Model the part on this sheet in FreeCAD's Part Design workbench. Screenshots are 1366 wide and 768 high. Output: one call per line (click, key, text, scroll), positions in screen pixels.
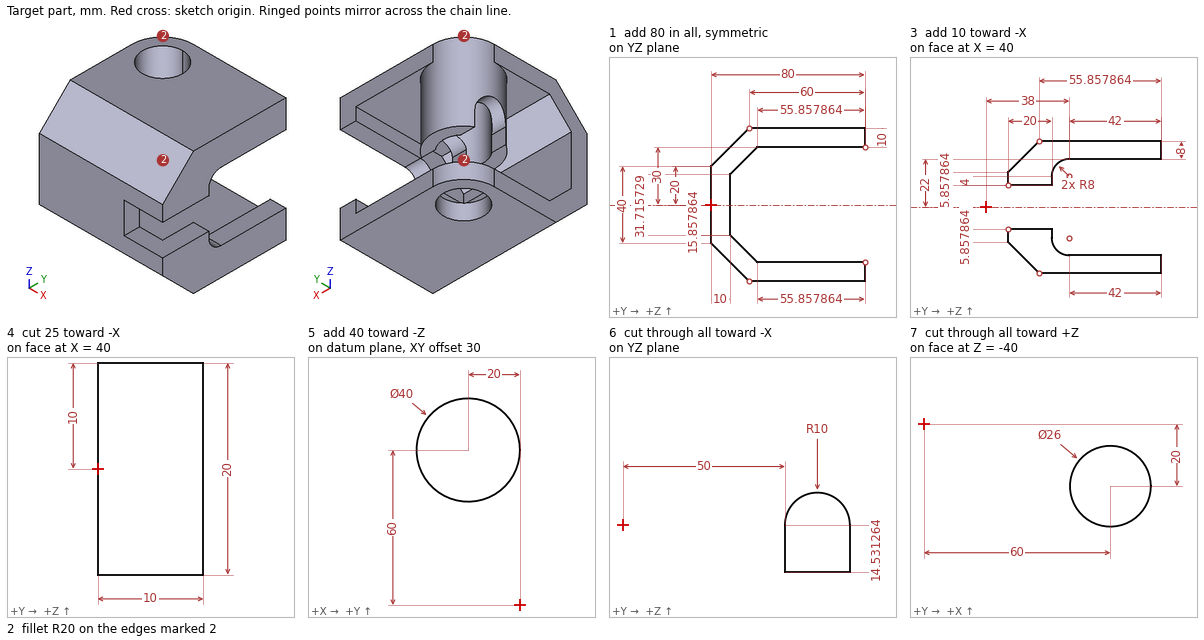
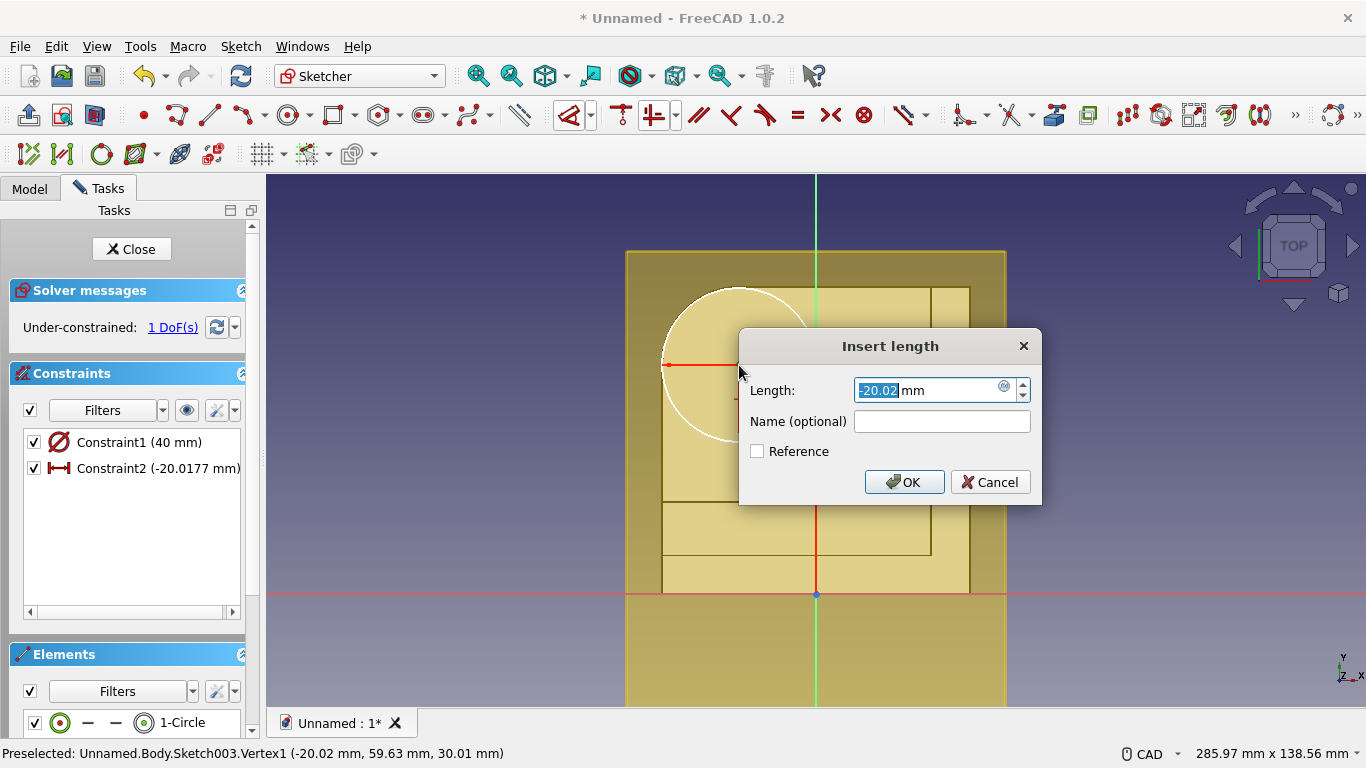
text(-20)
key(Return)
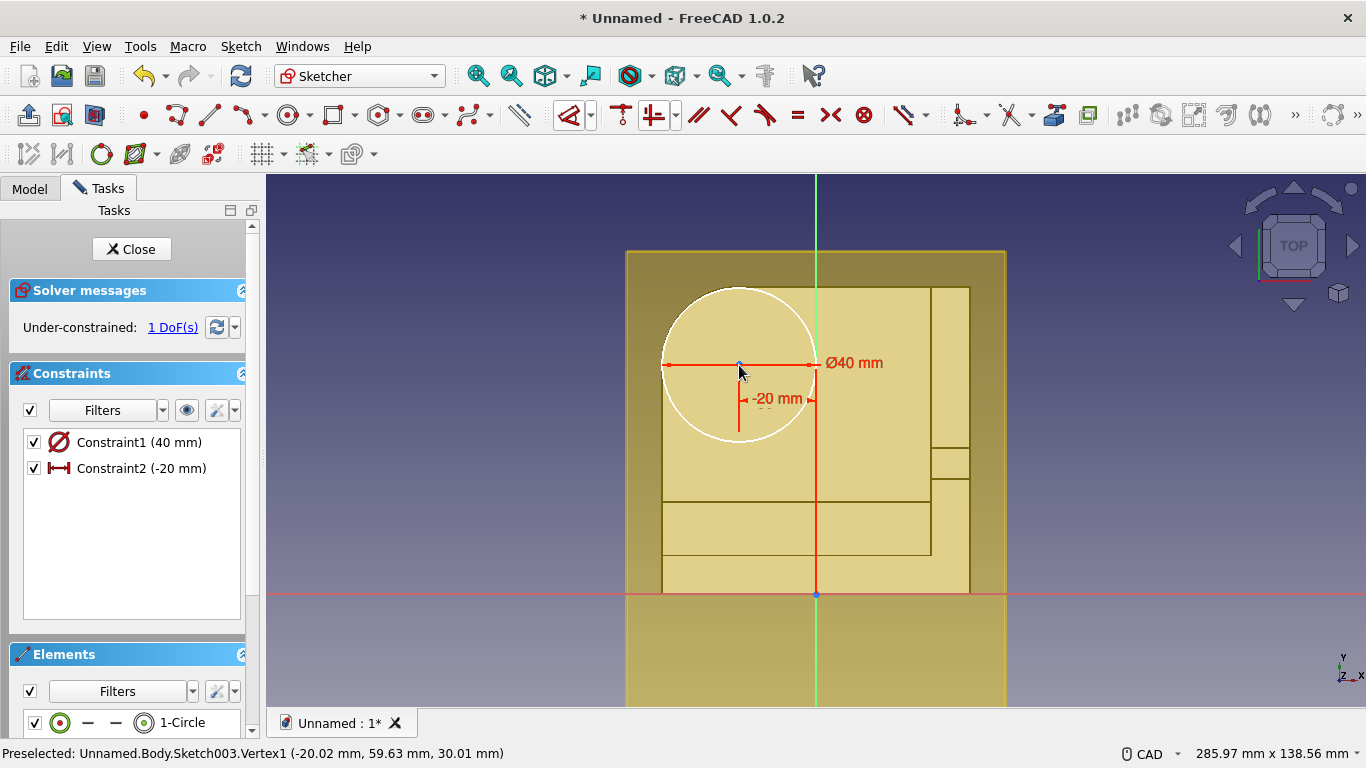
click(739, 365)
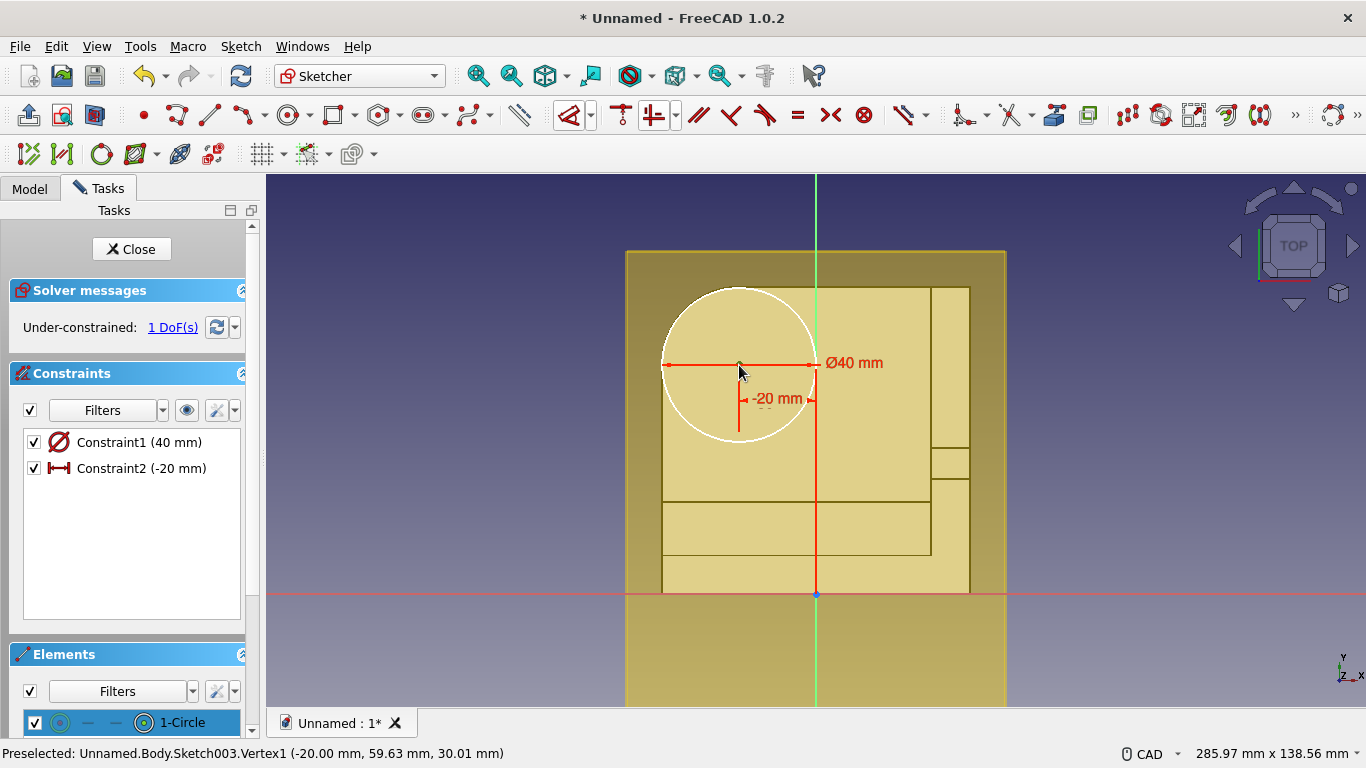
click(590, 116)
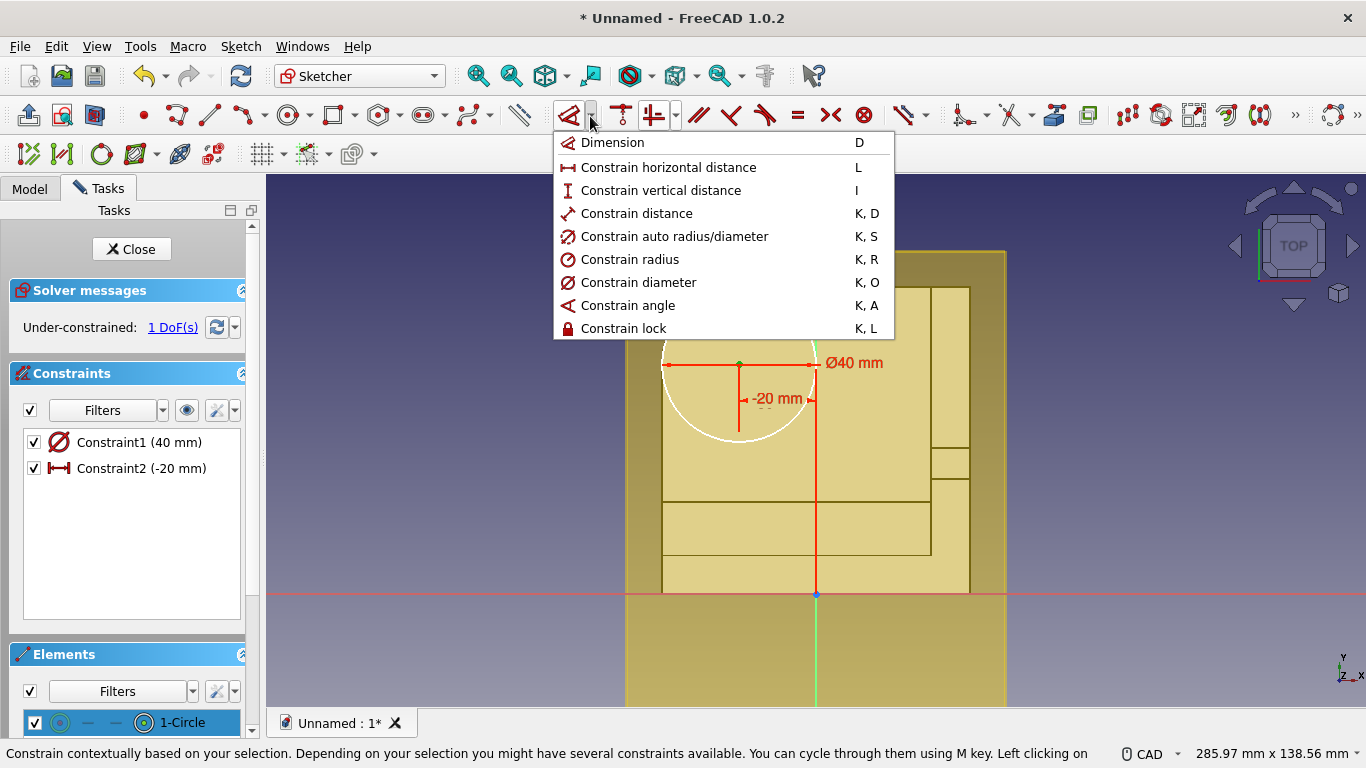
click(724, 190)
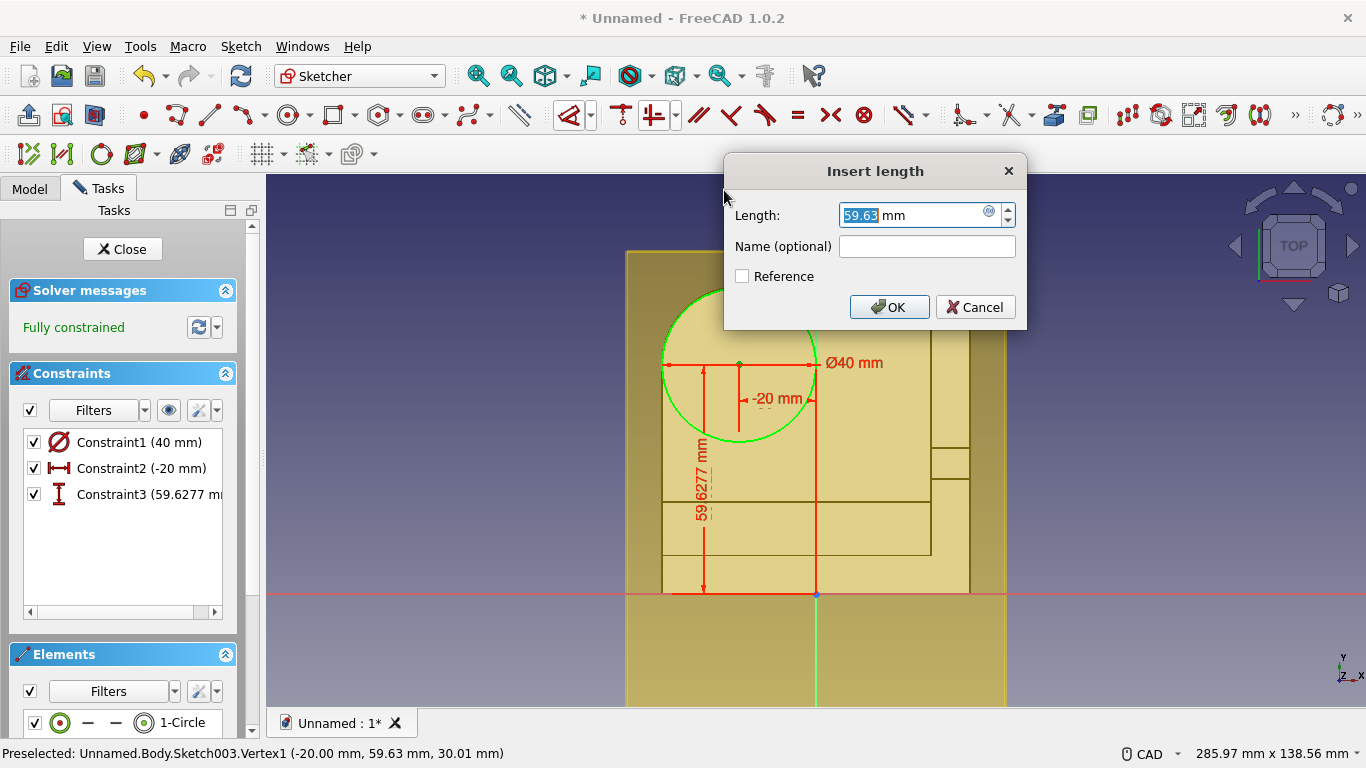
text(60)
key(Return)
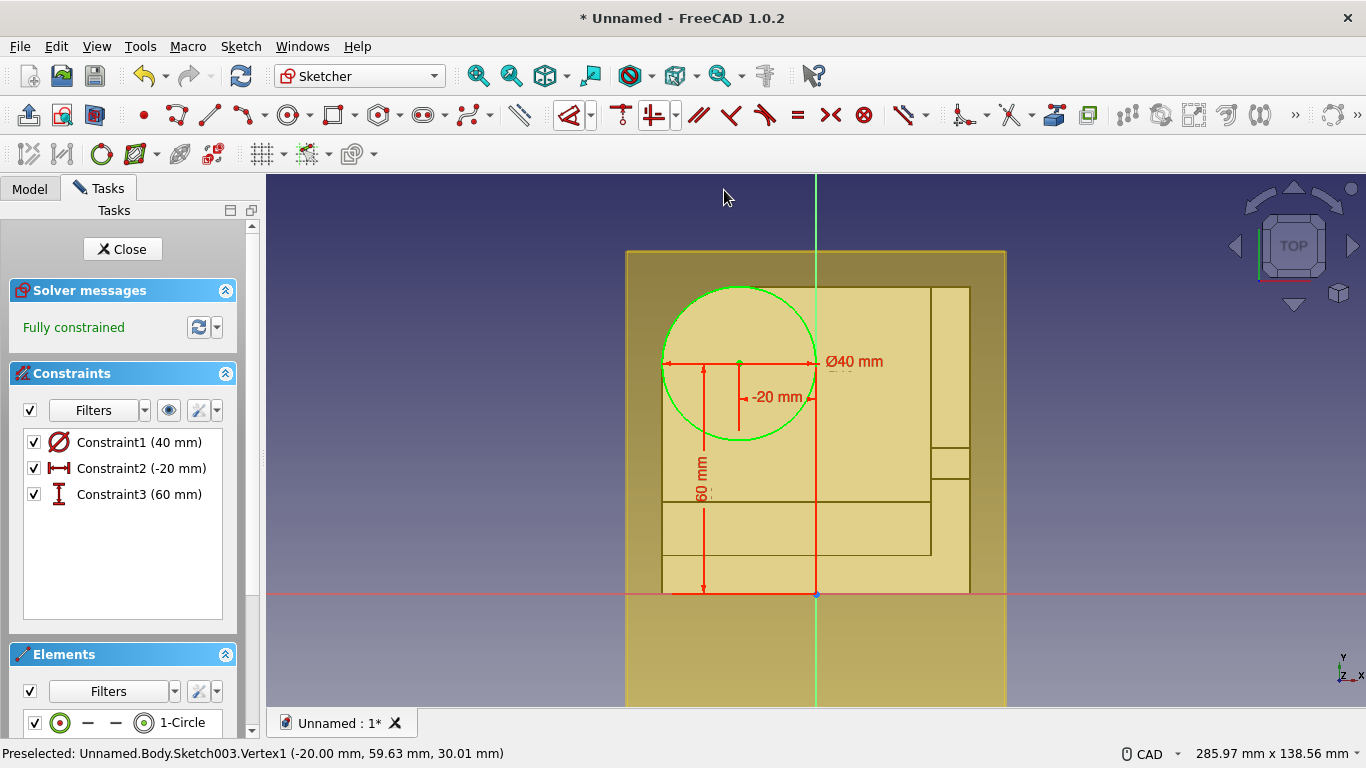
click(123, 249)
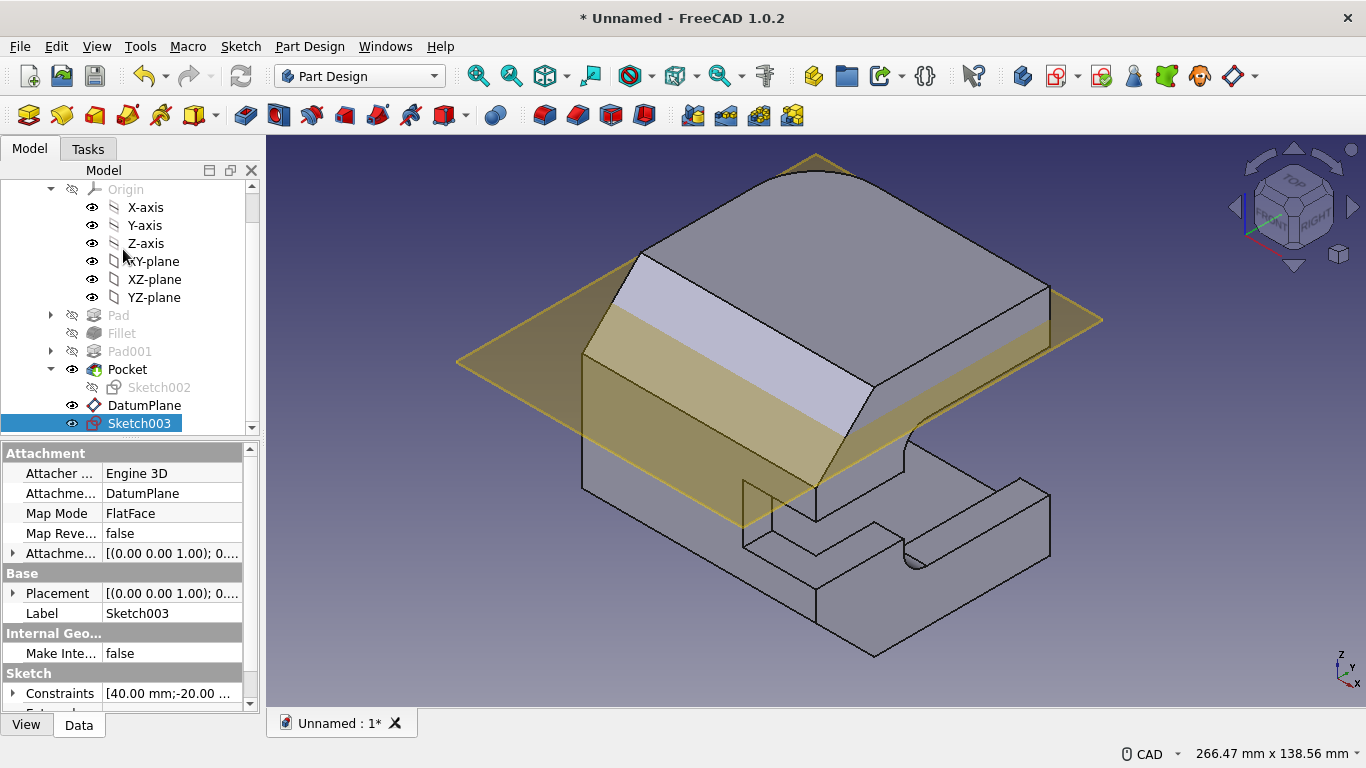
click(29, 116)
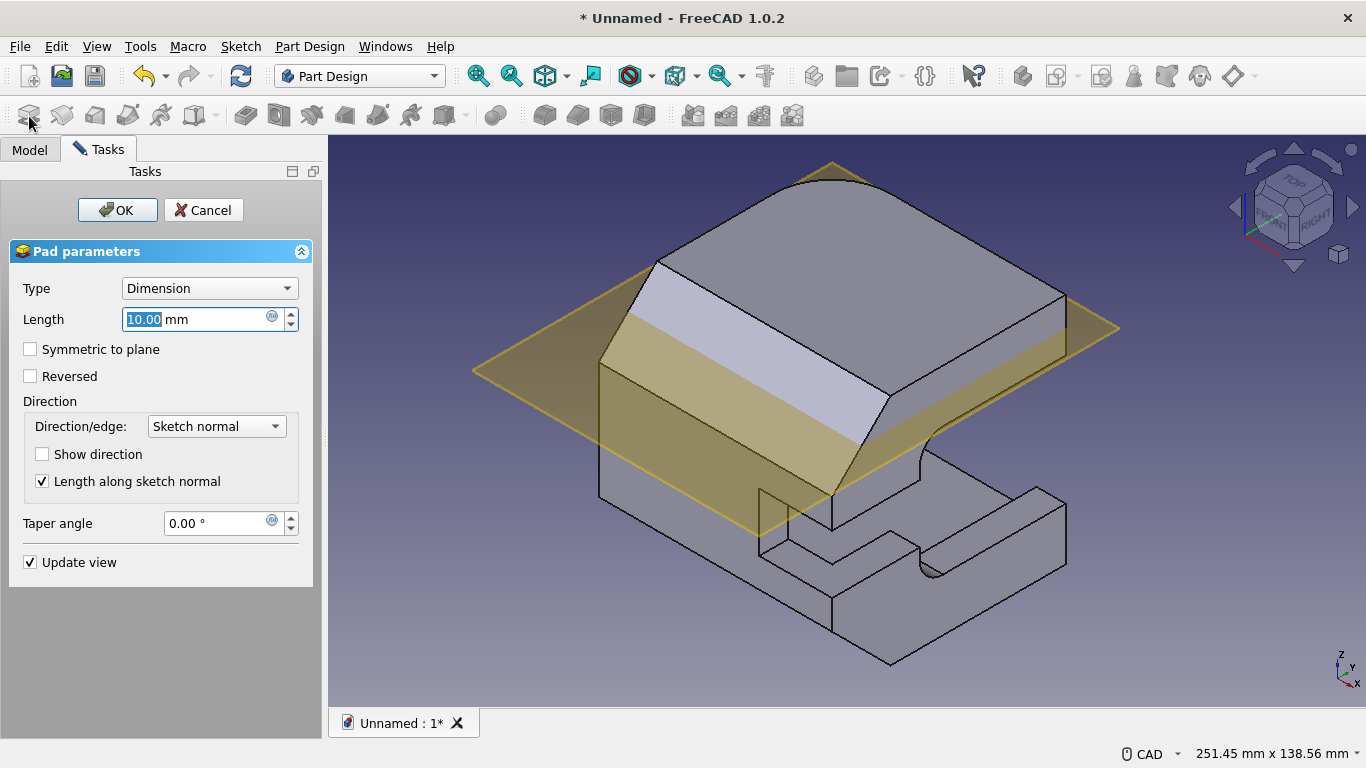
text(40)
key(Tab)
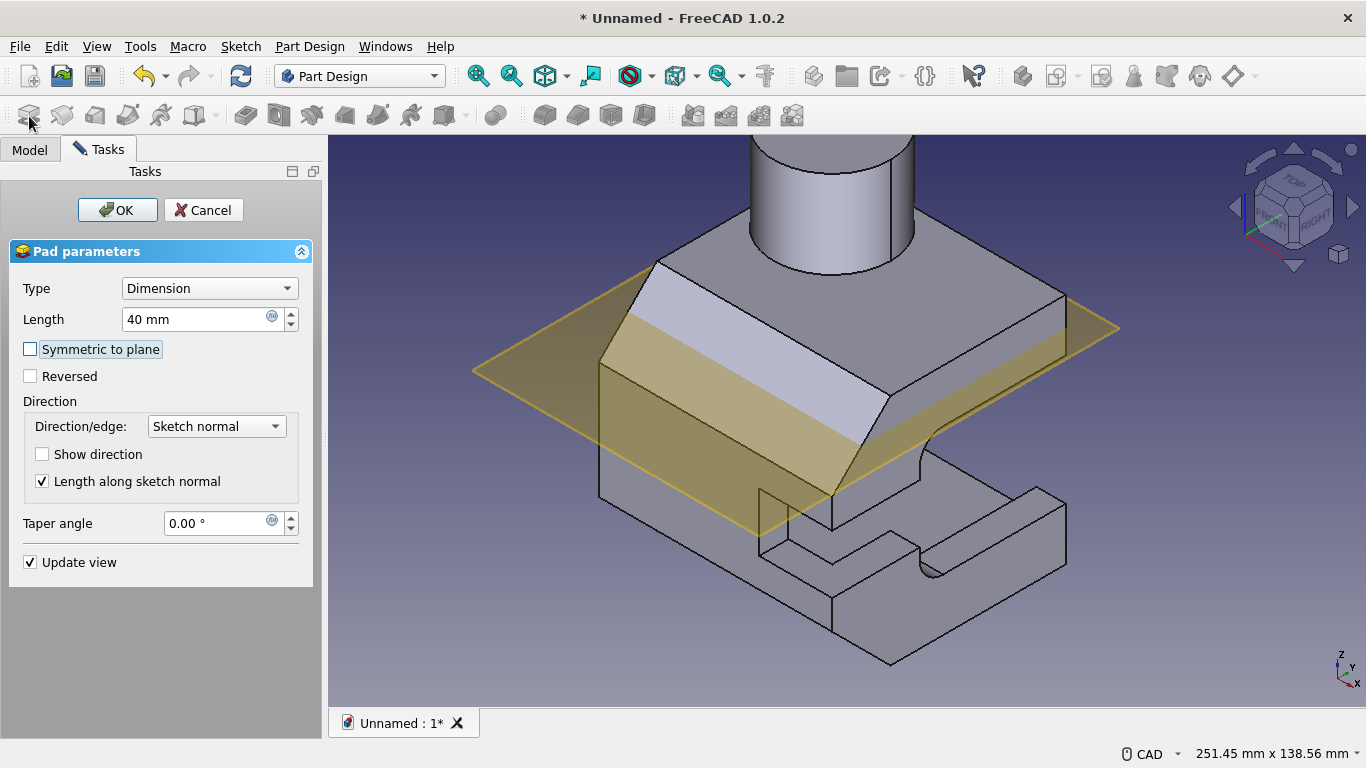
click(31, 376)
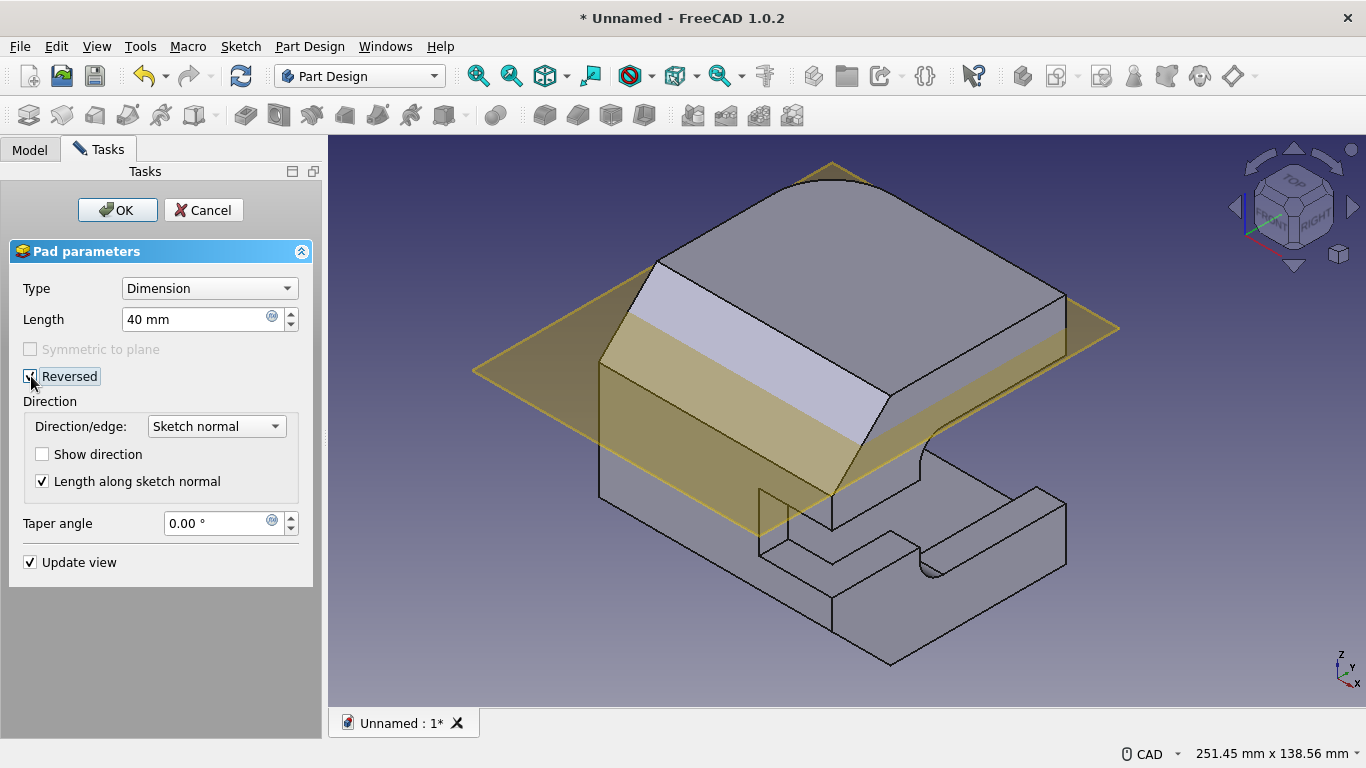
click(118, 210)